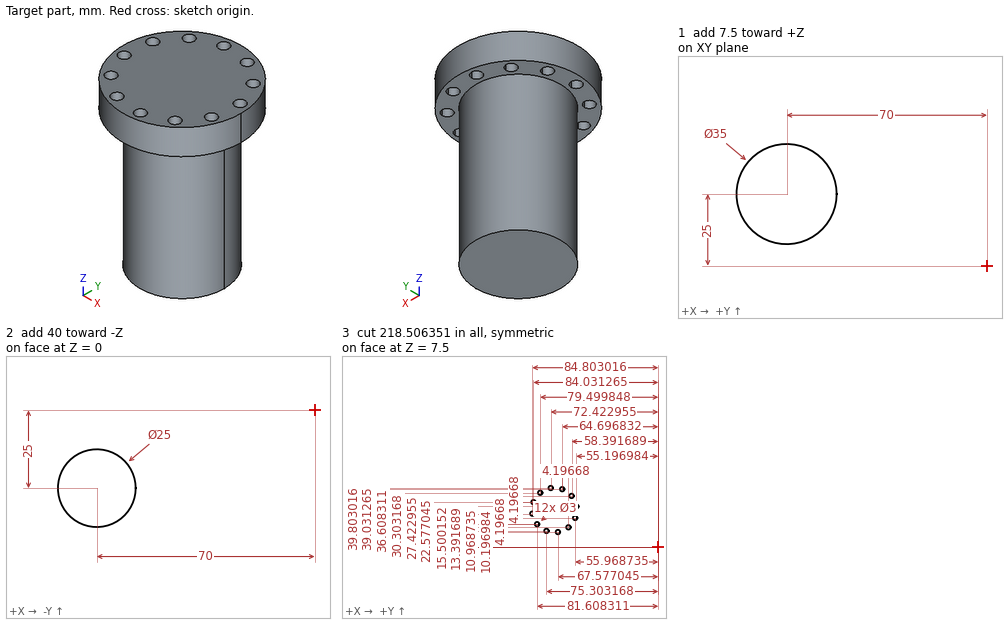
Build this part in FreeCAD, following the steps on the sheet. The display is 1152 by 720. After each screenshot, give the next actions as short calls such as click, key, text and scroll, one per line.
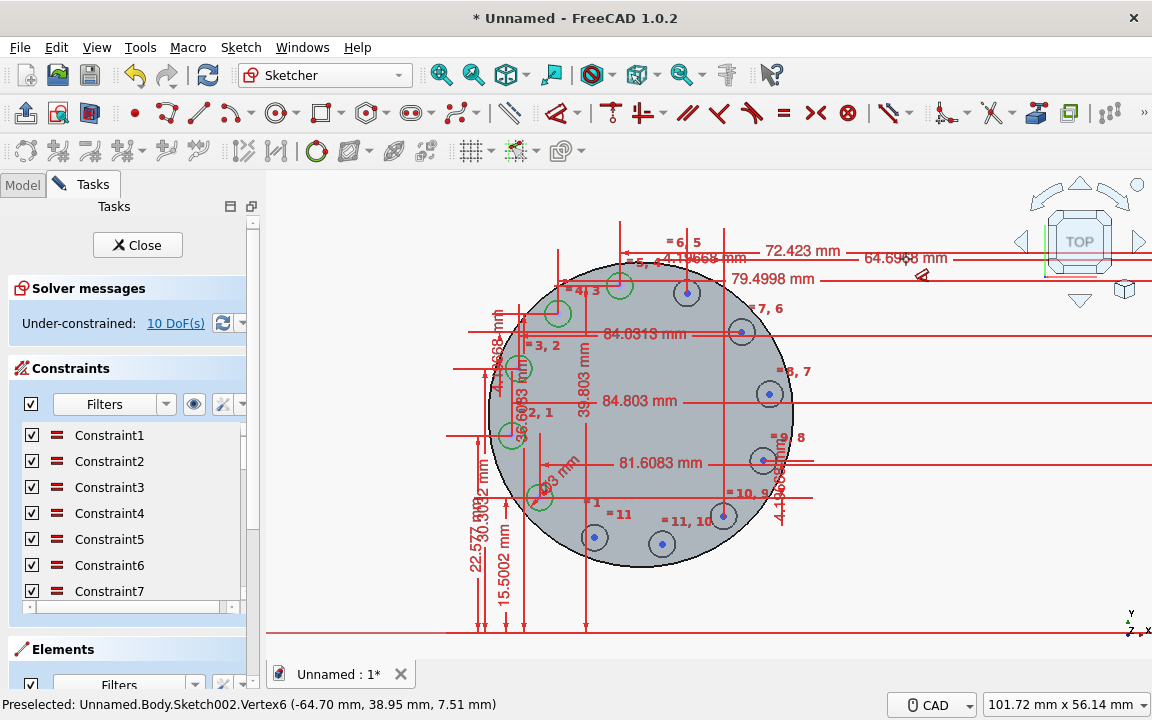
click(687, 293)
click(653, 580)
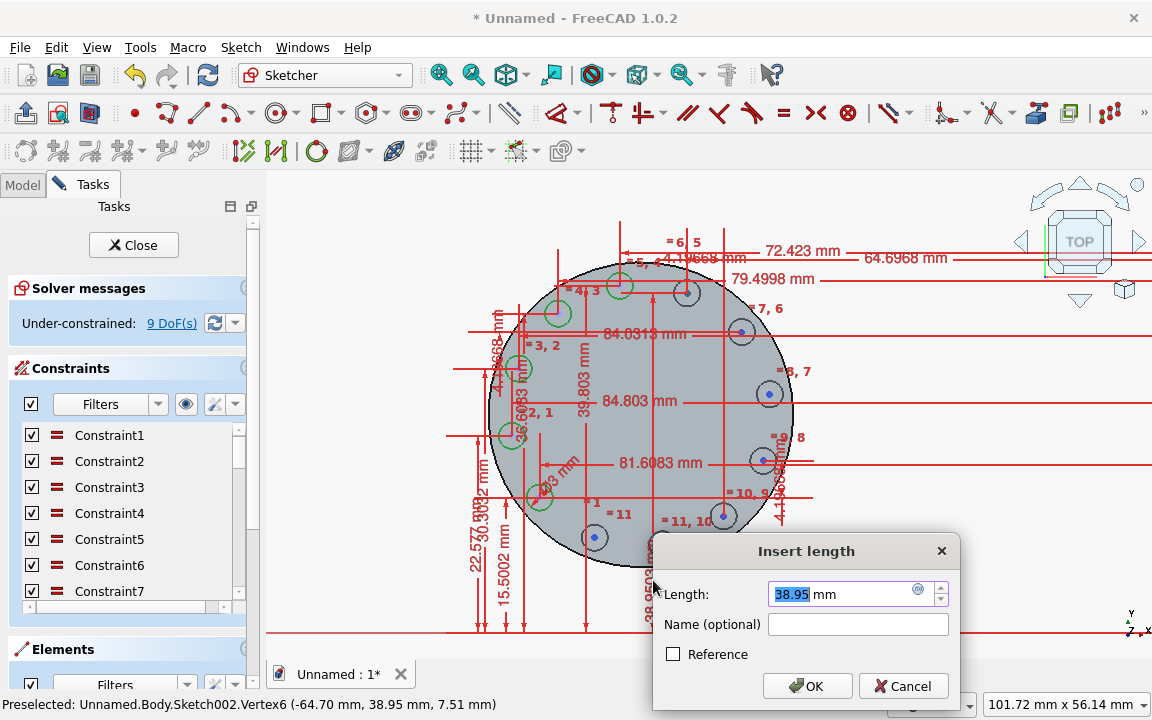
text(39.031265)
key(Return)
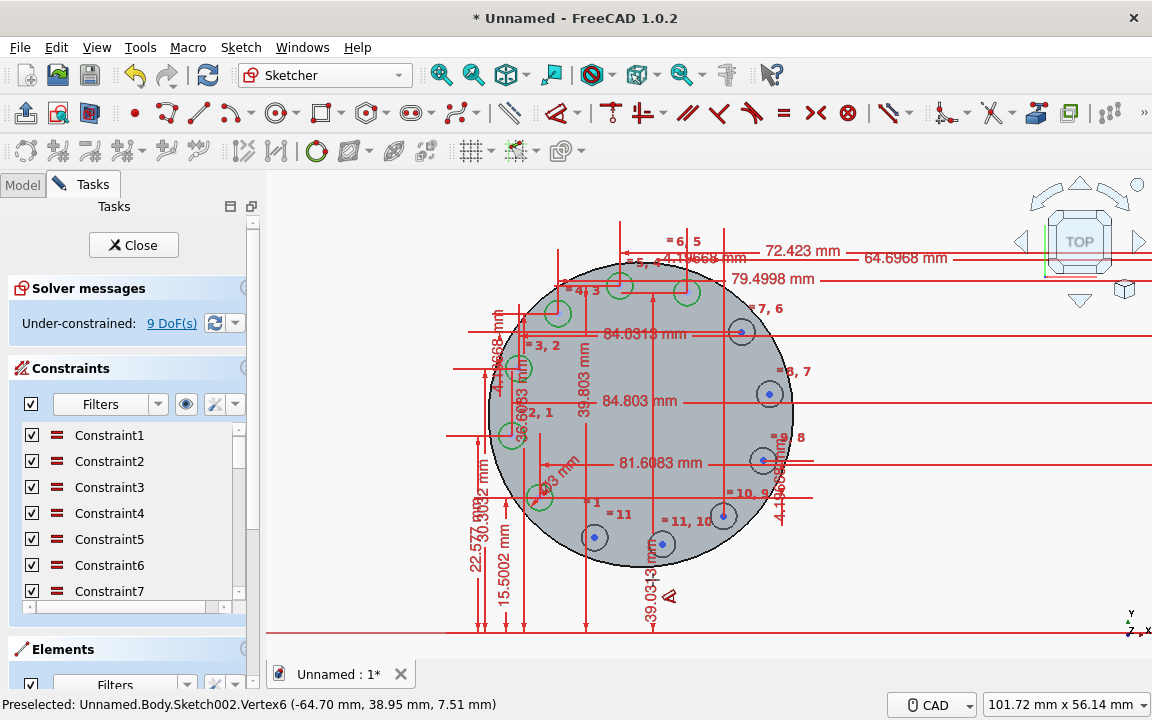
click(742, 332)
click(864, 298)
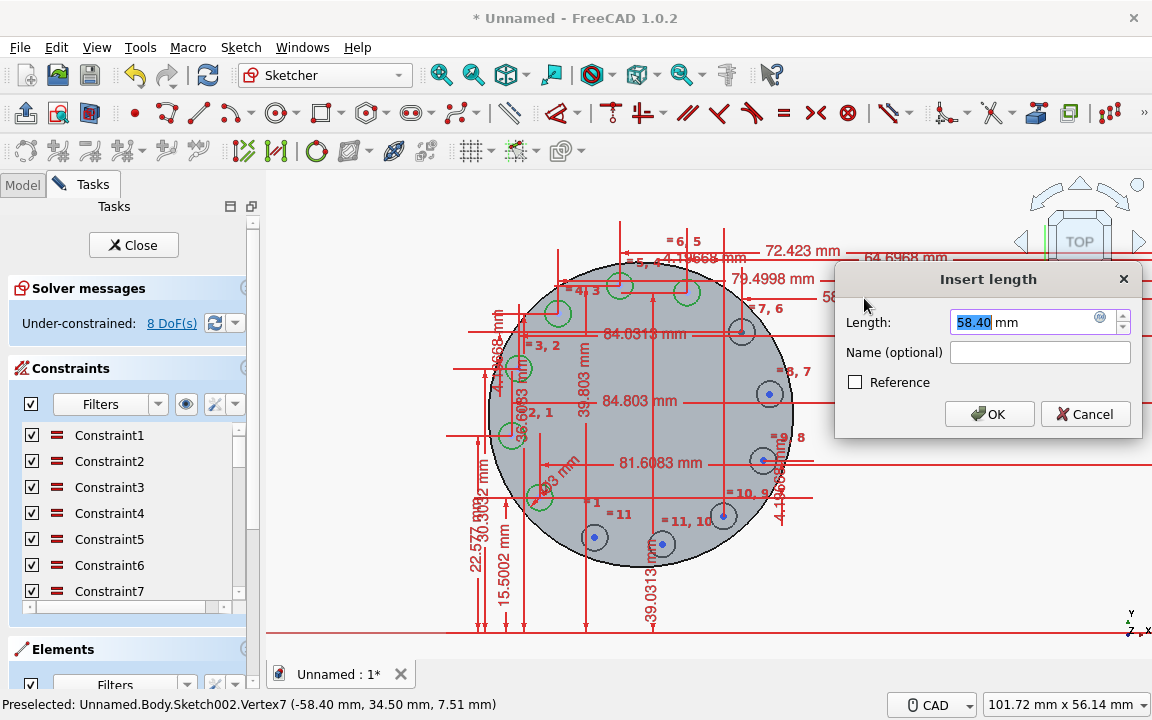
text(58.391689)
key(Return)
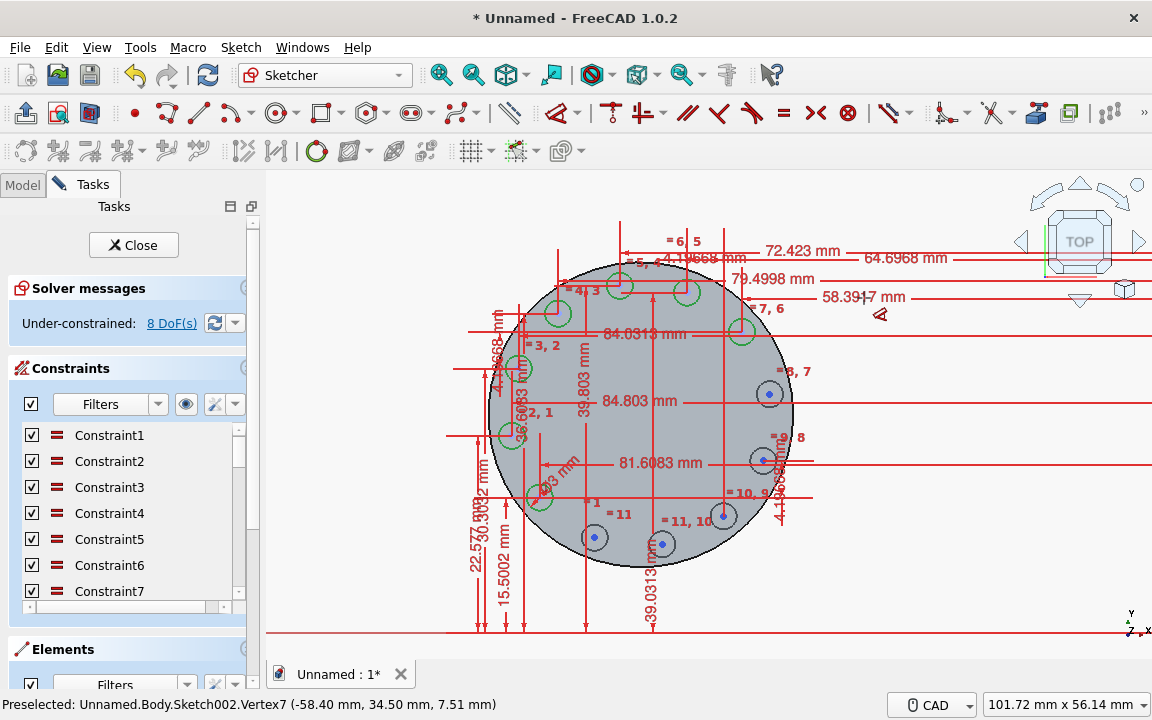
click(770, 394)
click(878, 360)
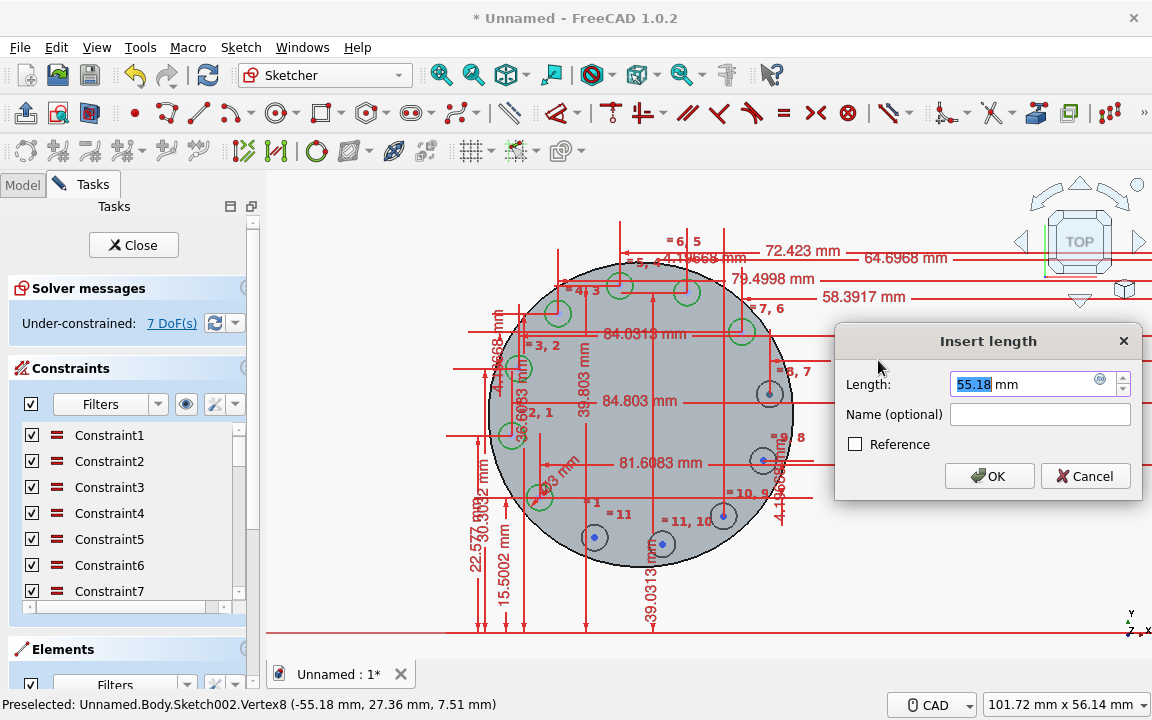
text(55.196984)
key(Return)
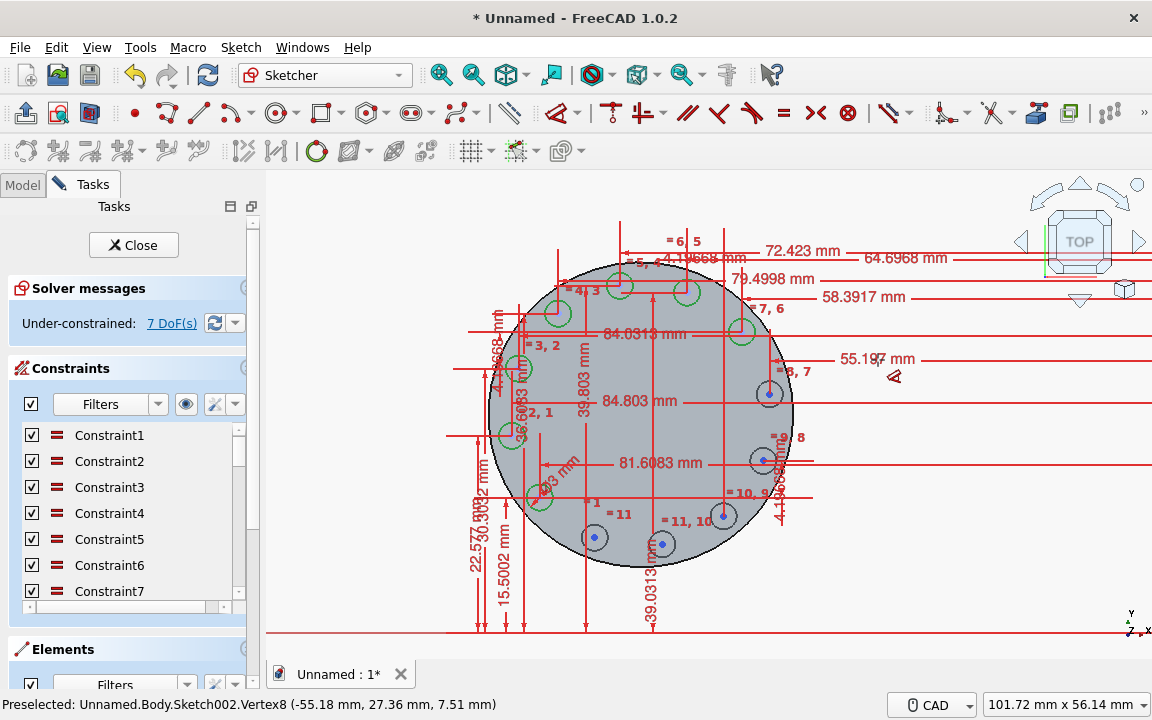
click(770, 394)
click(736, 458)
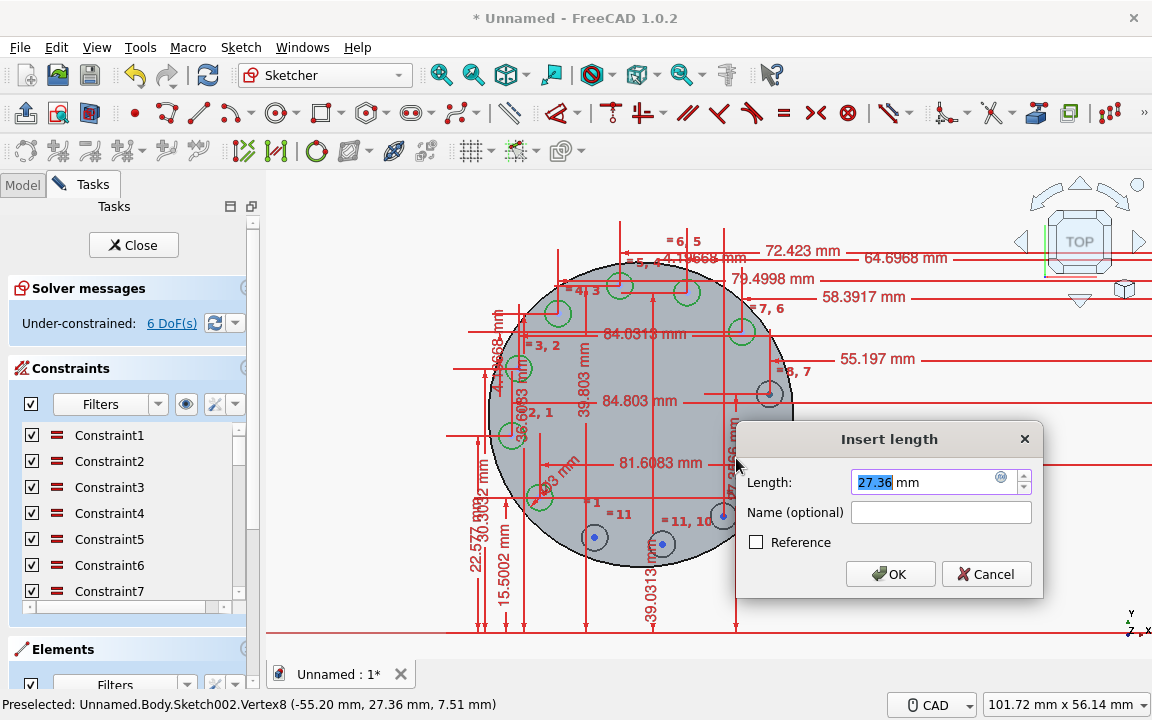
text(27.422955)
key(Return)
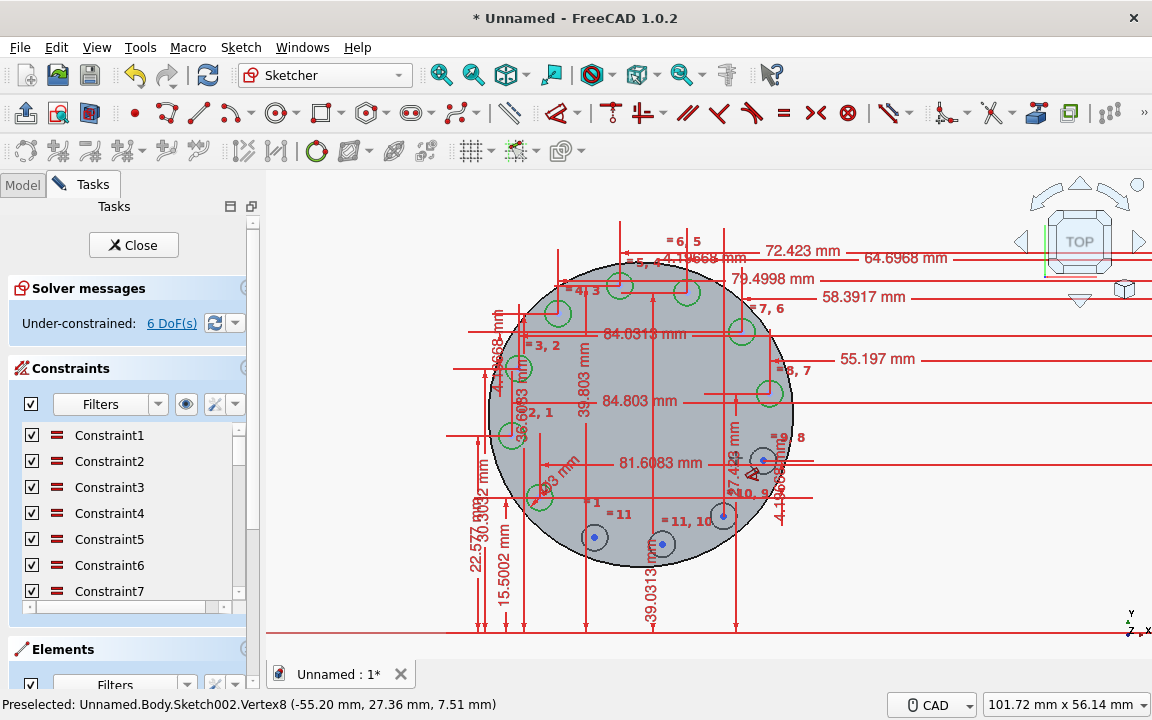
click(763, 461)
click(875, 427)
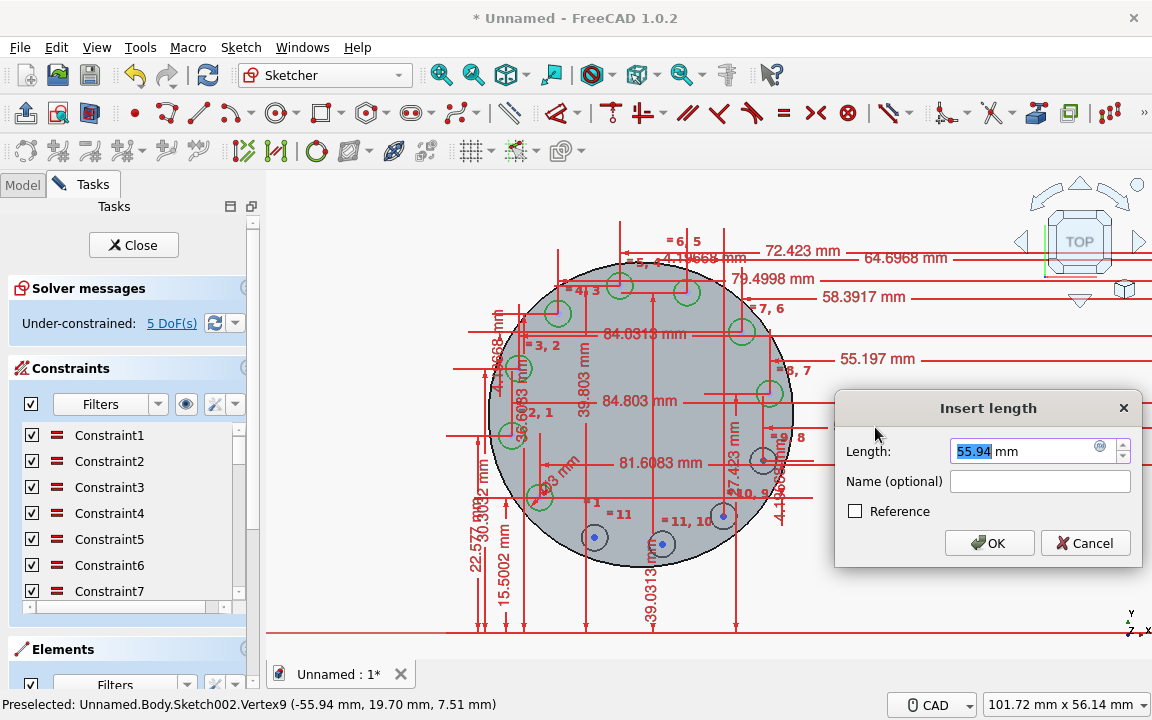
text(55.968735)
key(Return)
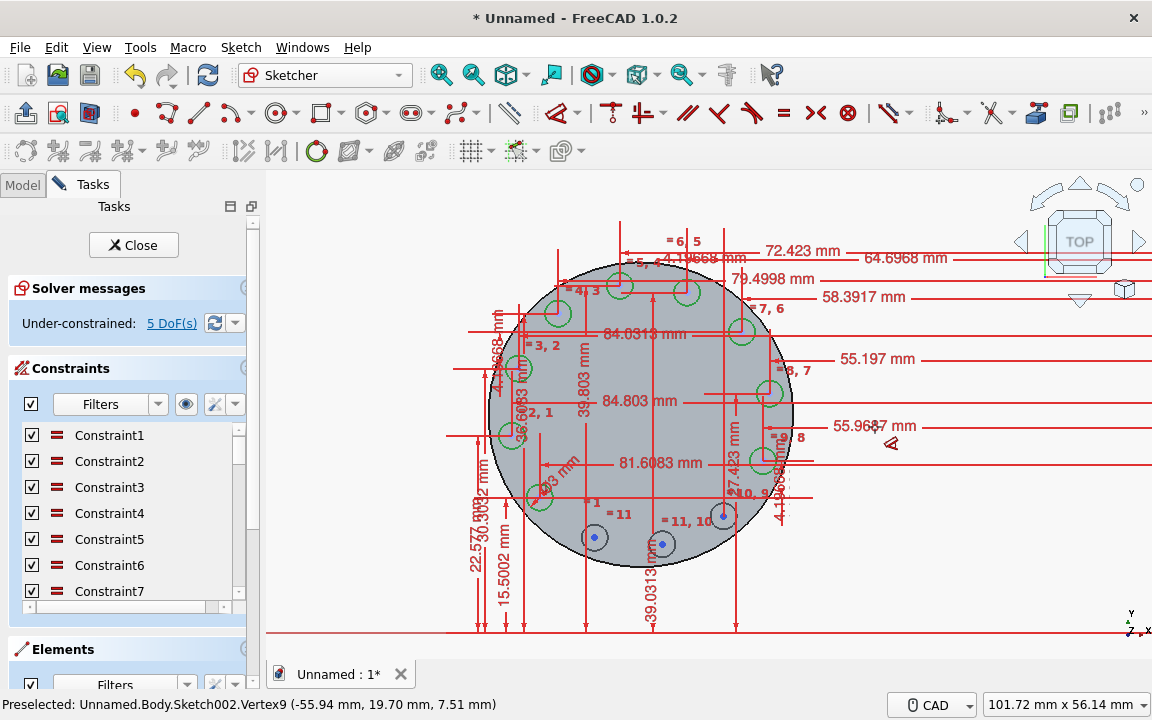
click(724, 516)
click(690, 547)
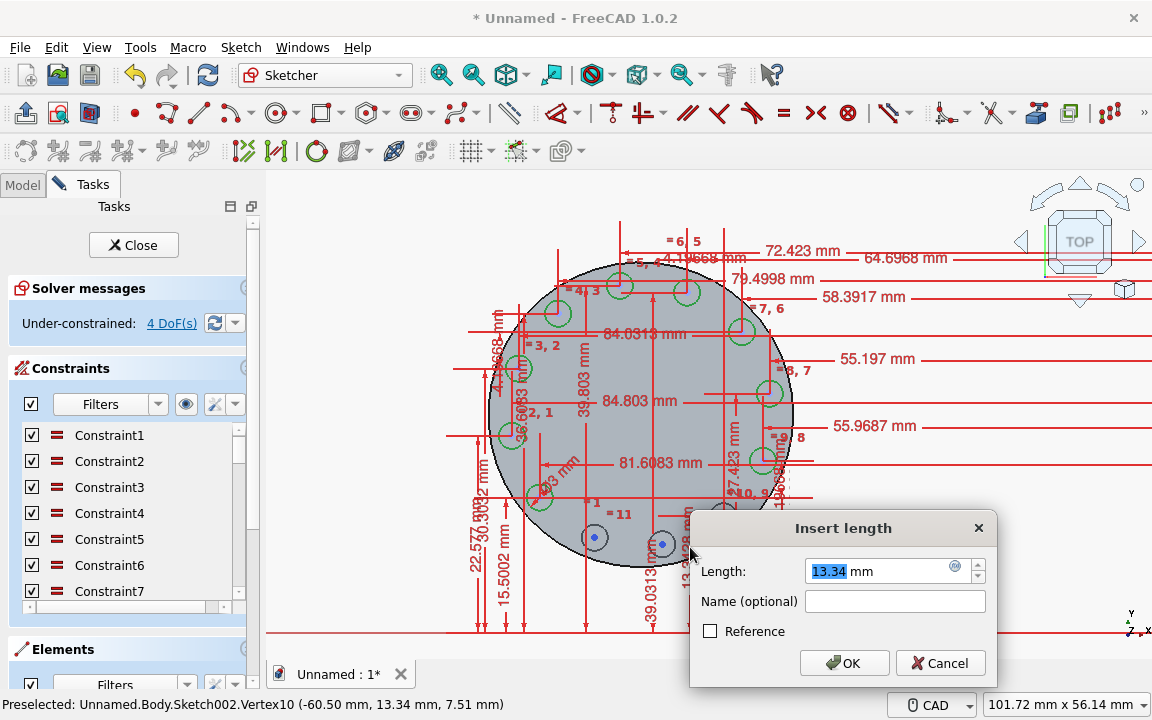
text(13.391689)
key(Return)